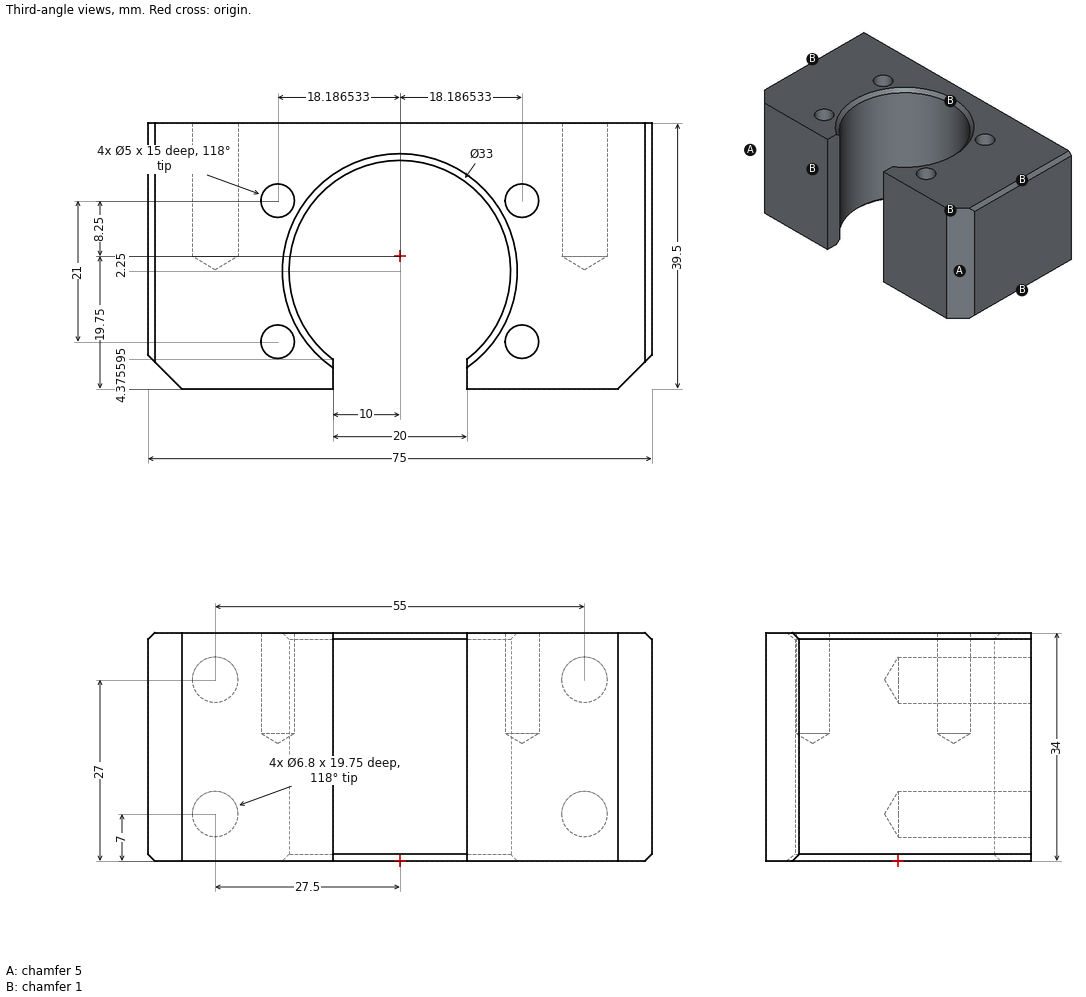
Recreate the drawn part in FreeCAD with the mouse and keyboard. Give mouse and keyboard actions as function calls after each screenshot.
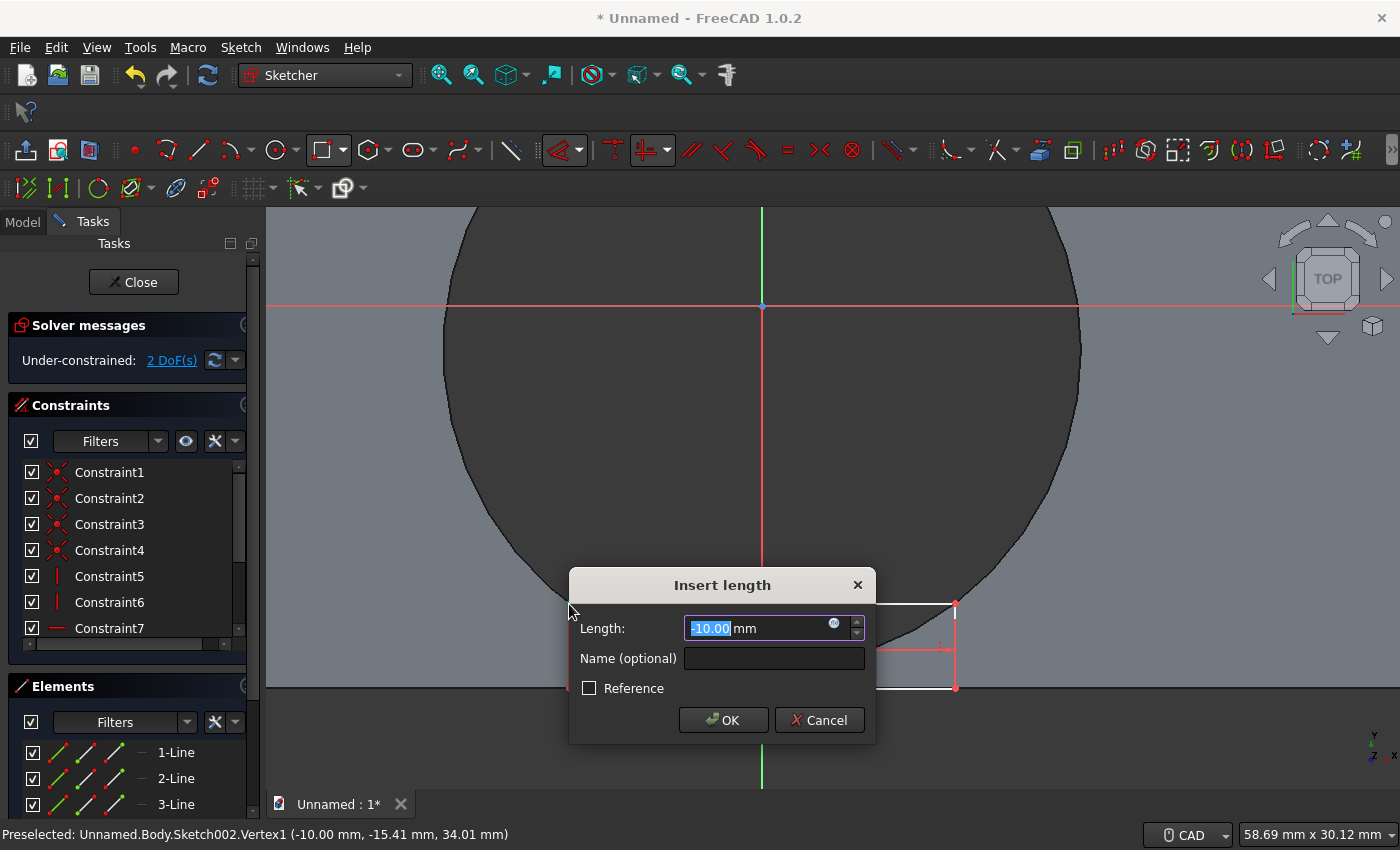
text(-10)
key(Return)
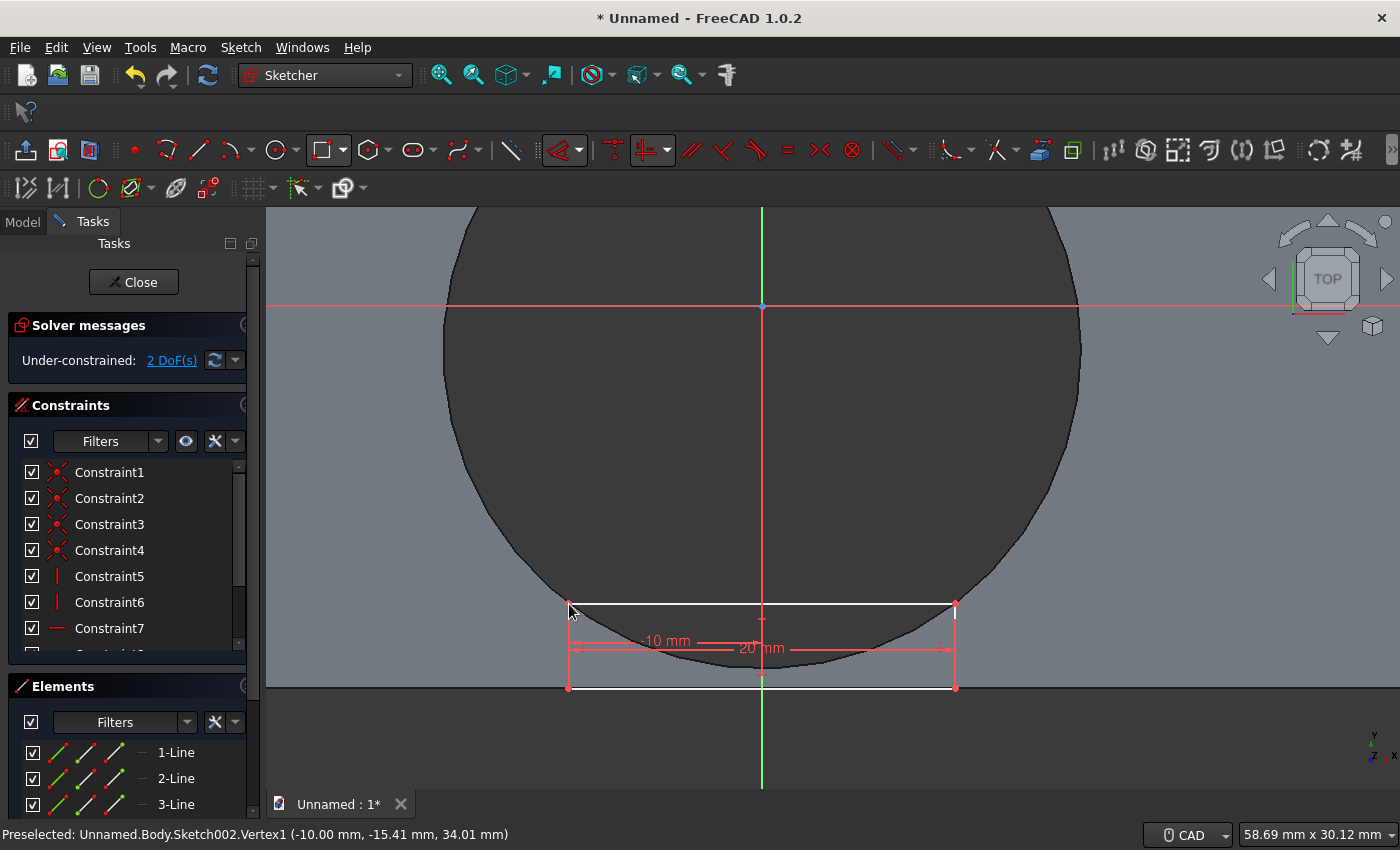
click(569, 689)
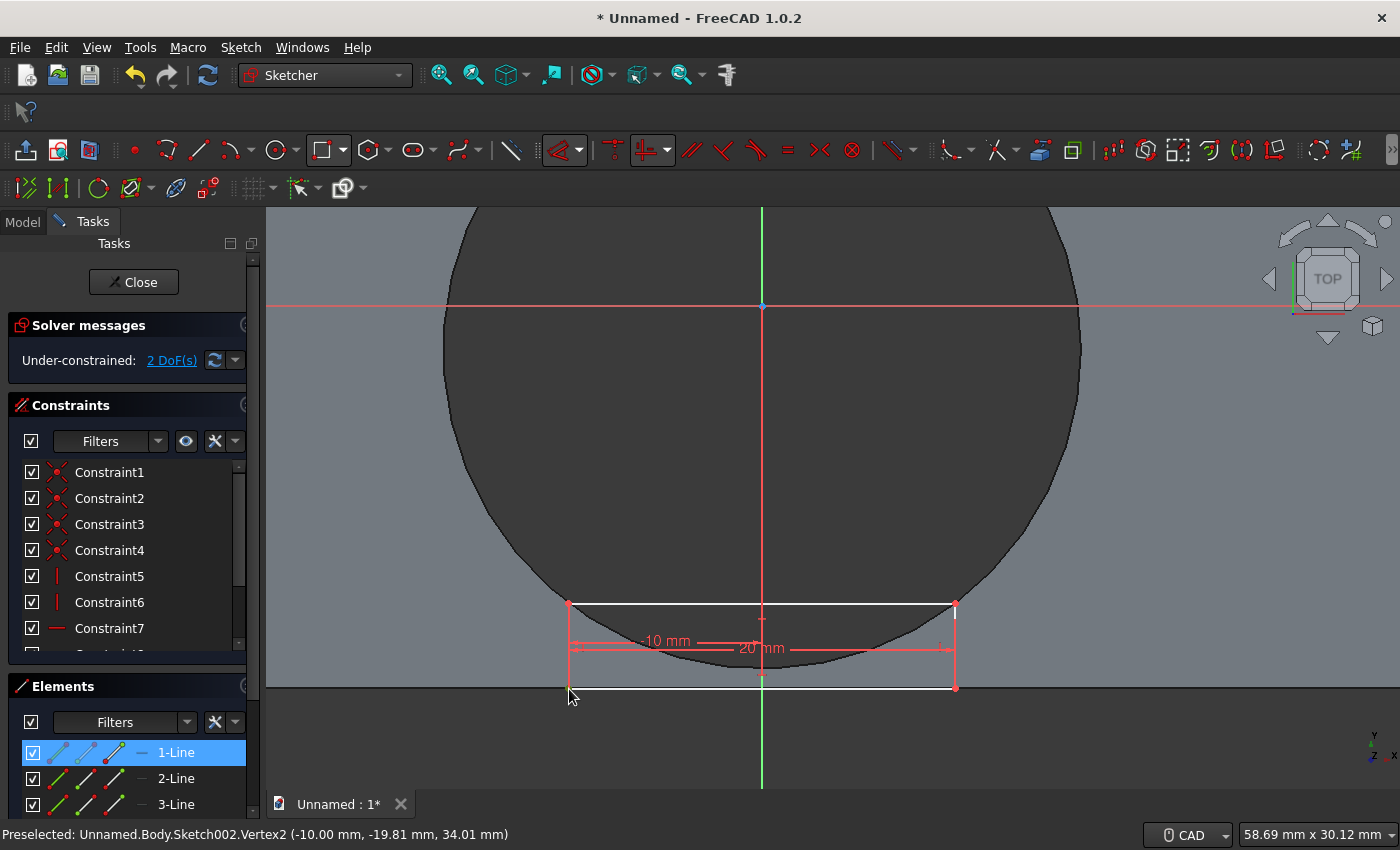
key(i)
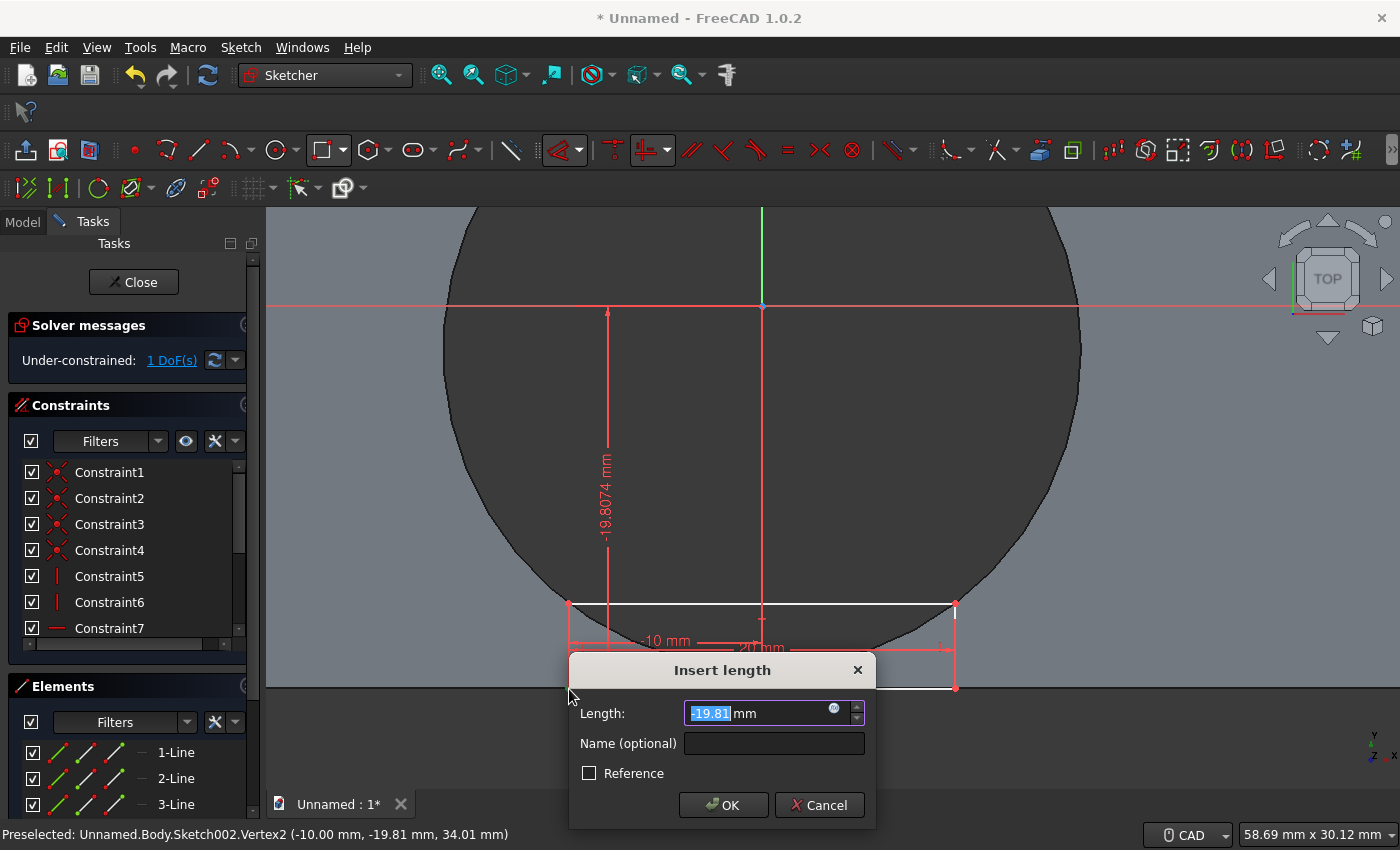
text(-19.75)
key(Return)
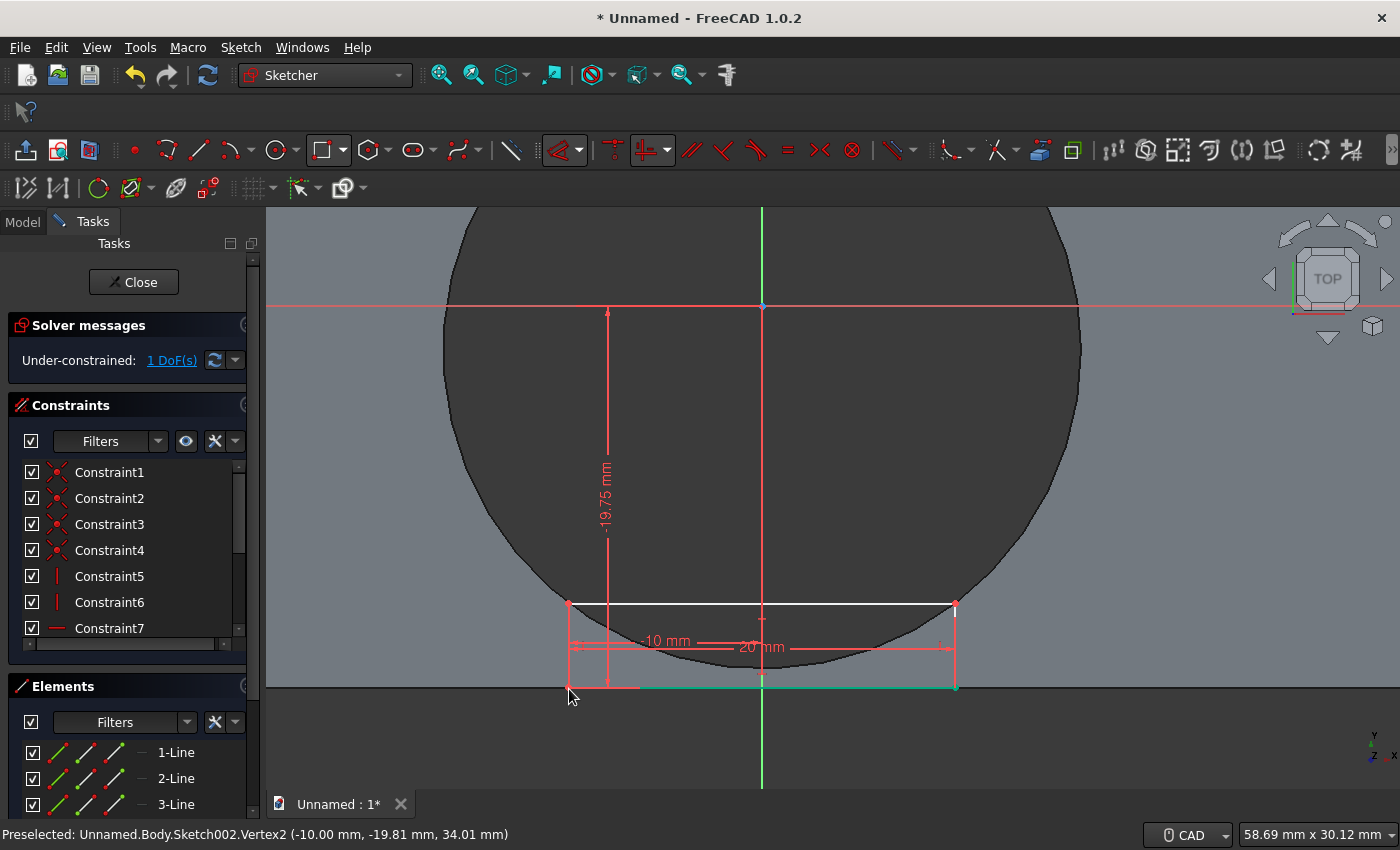
click(569, 629)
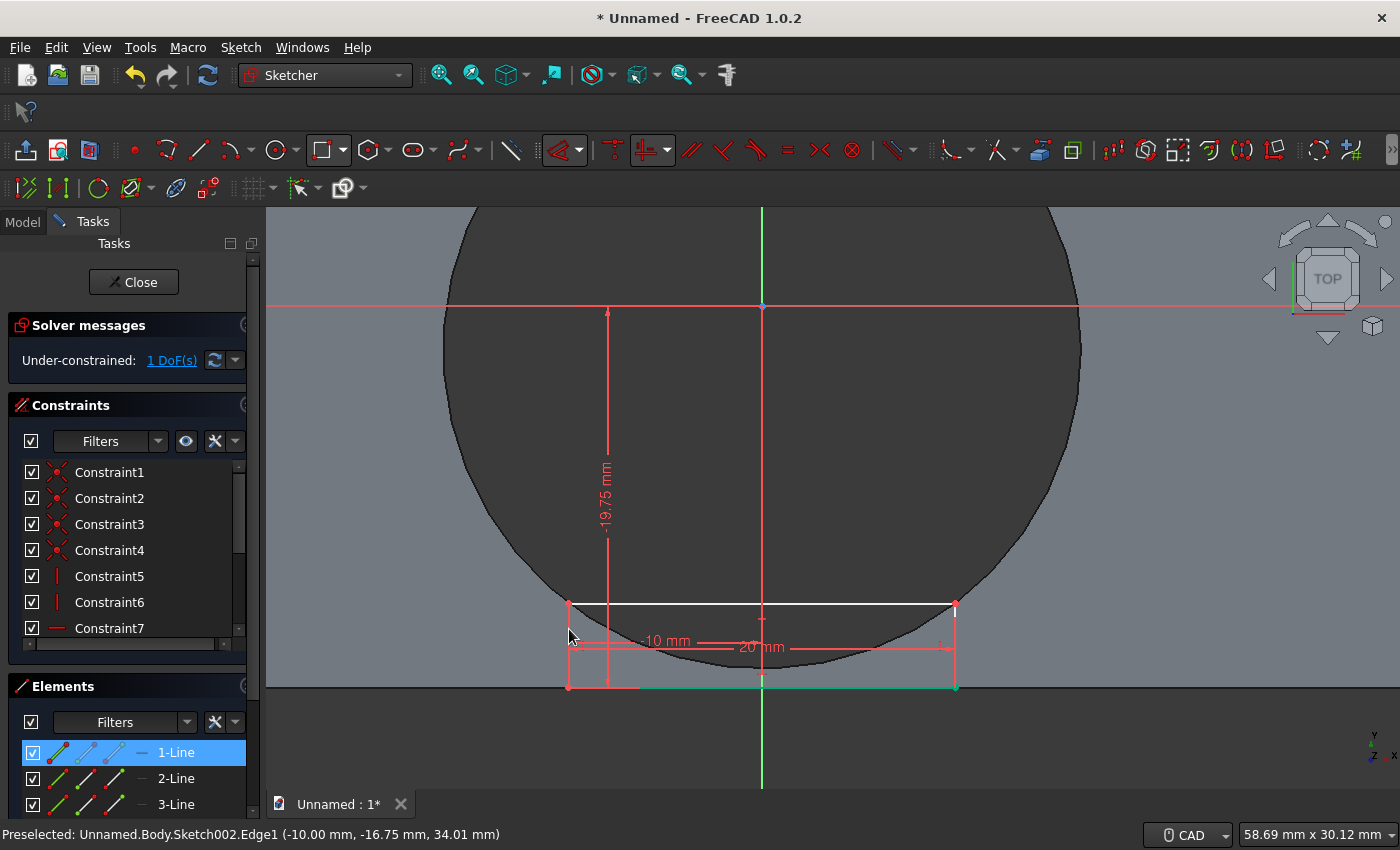
key(i)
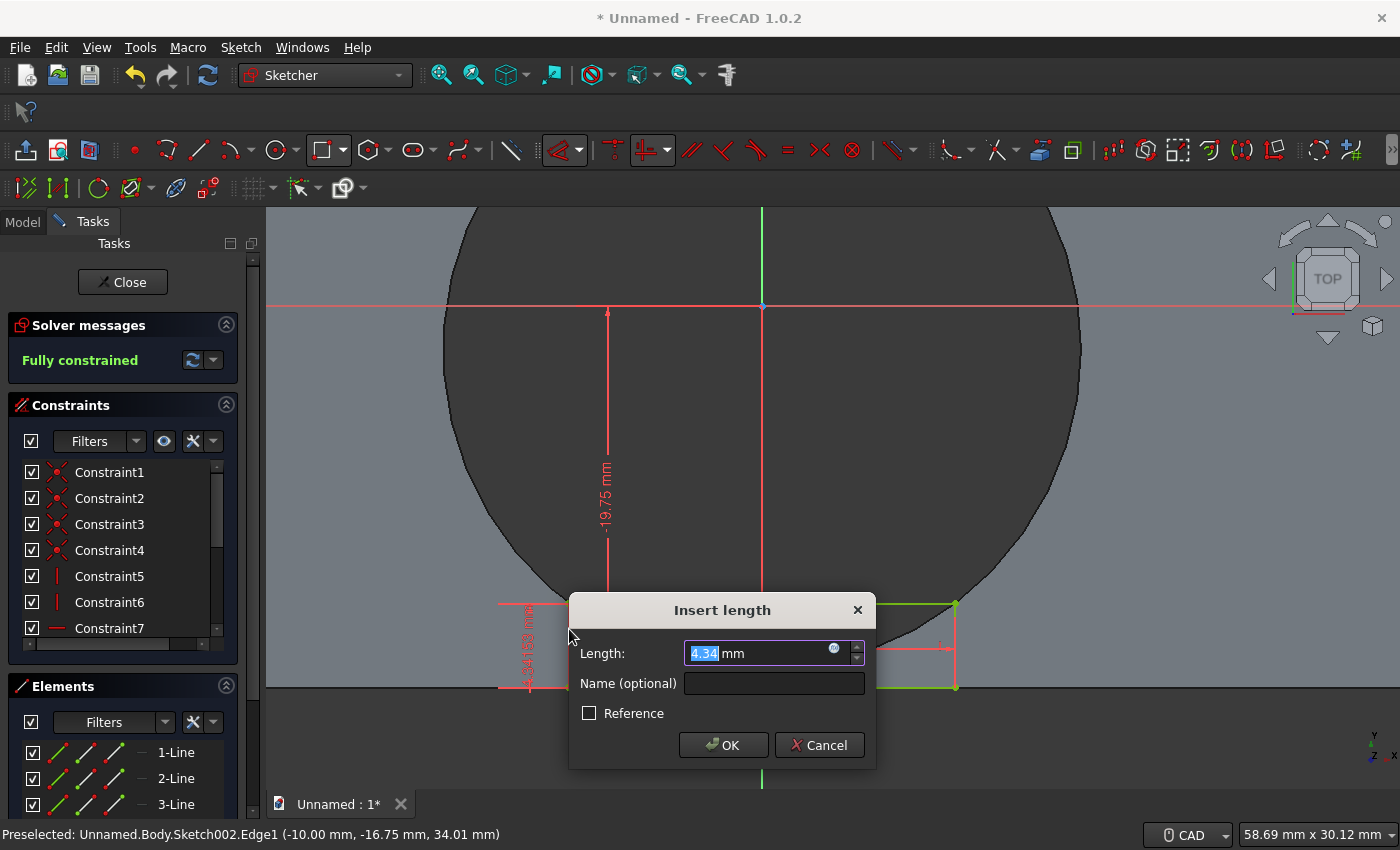
text(4.375595)
key(Return)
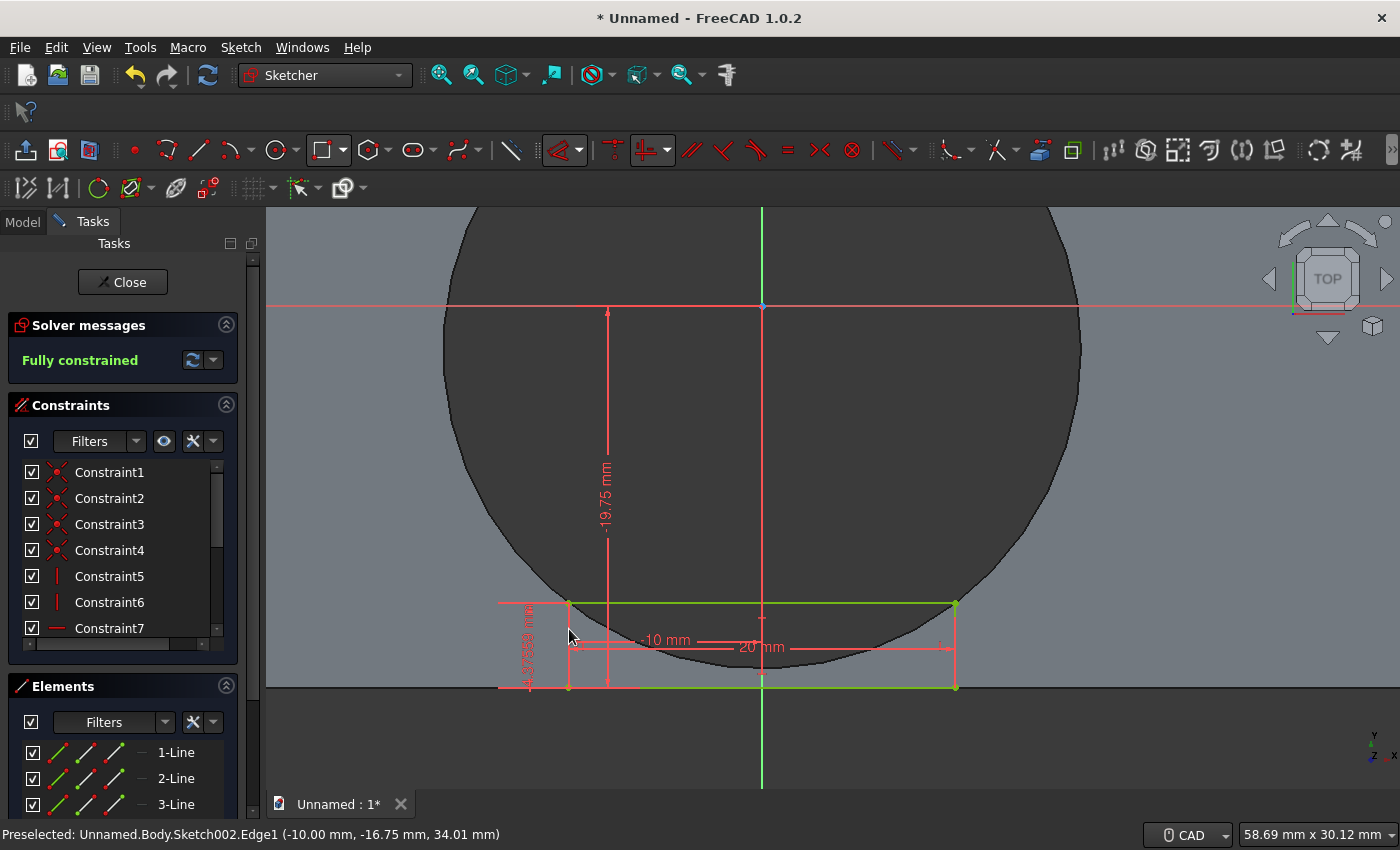
click(123, 282)